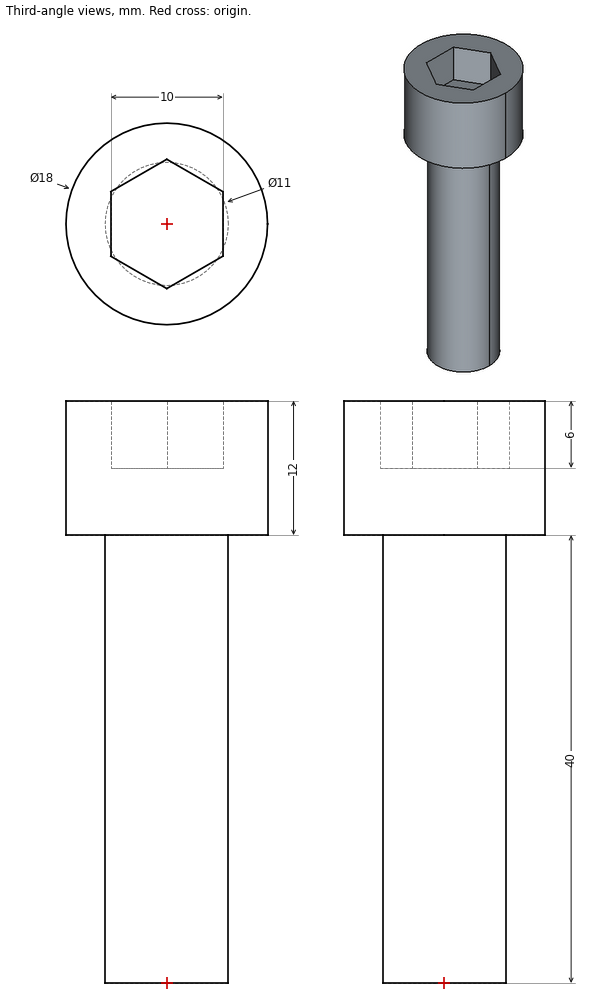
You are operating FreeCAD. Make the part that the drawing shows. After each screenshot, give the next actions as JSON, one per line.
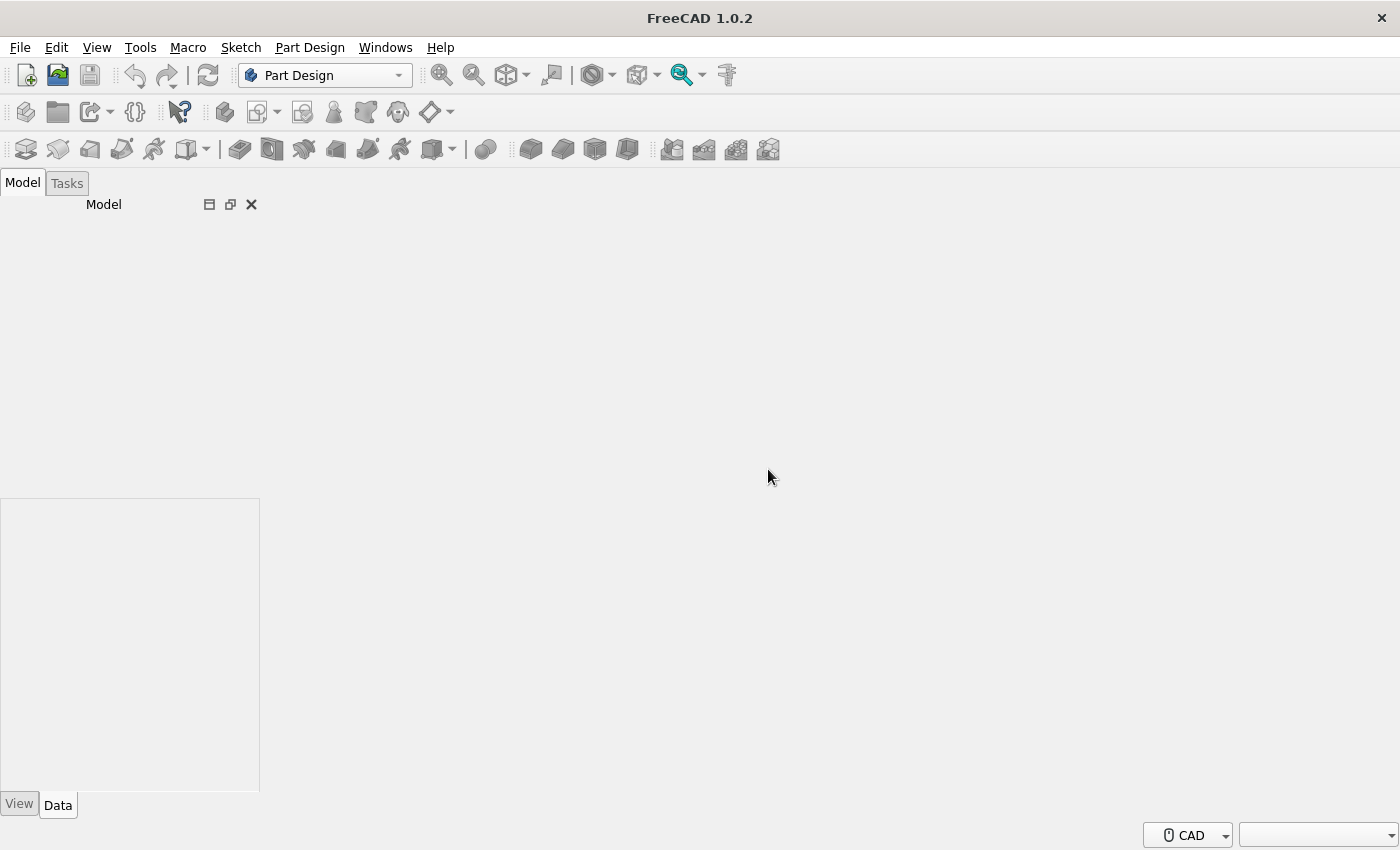
{"action": "left_click", "coordinate": [26, 76]}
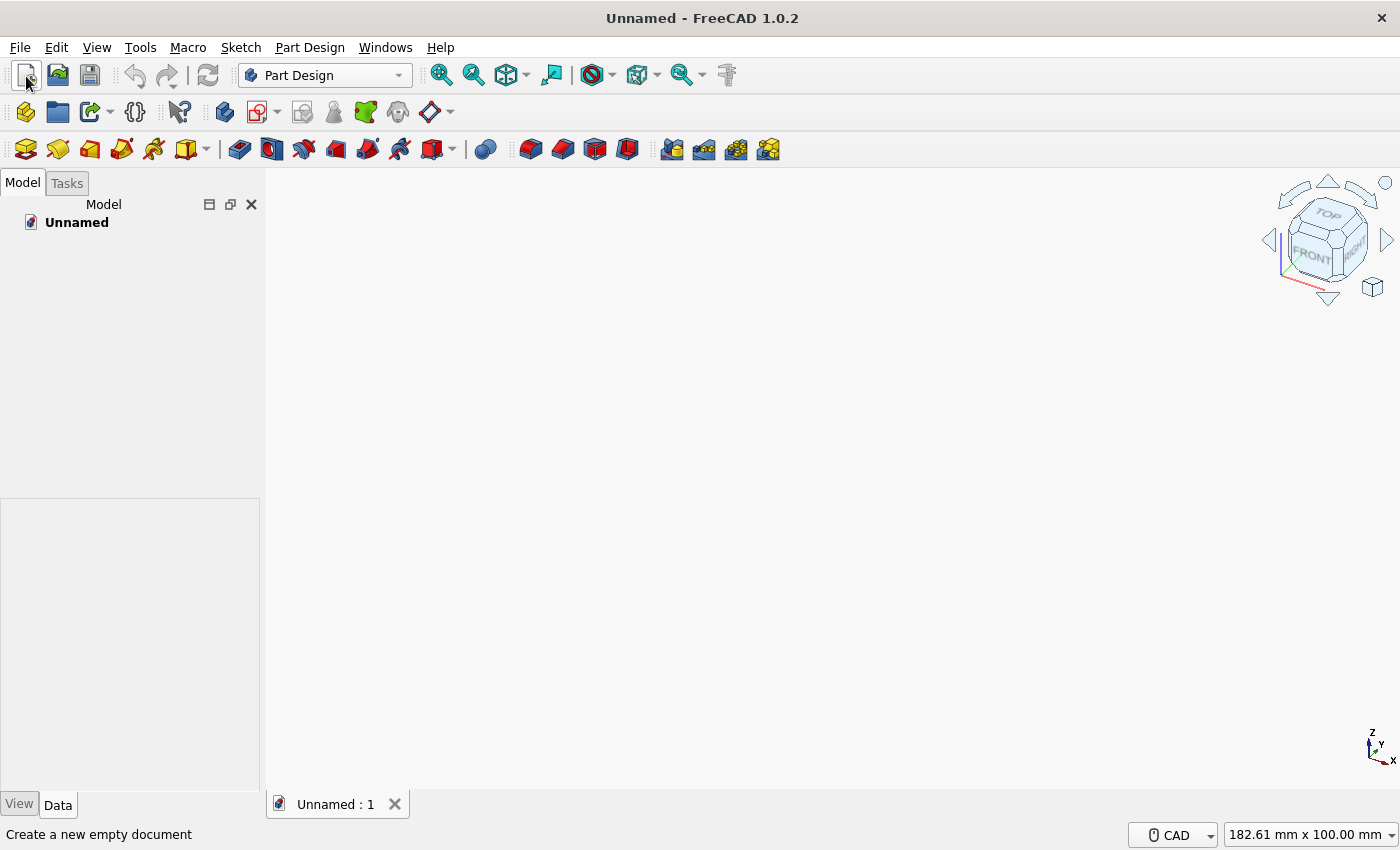
{"action": "left_click", "coordinate": [258, 112]}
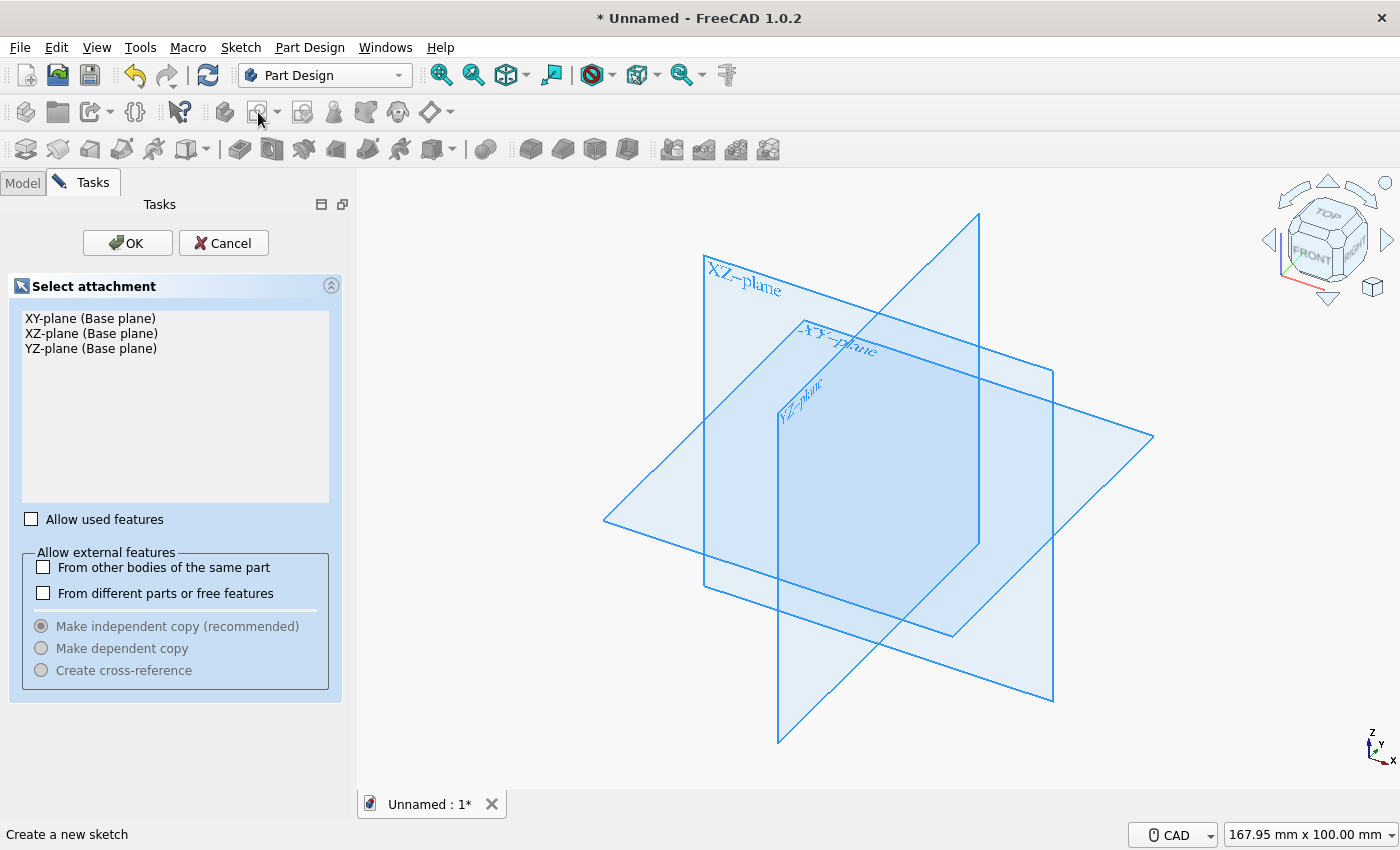
{"action": "left_click", "coordinate": [82, 318]}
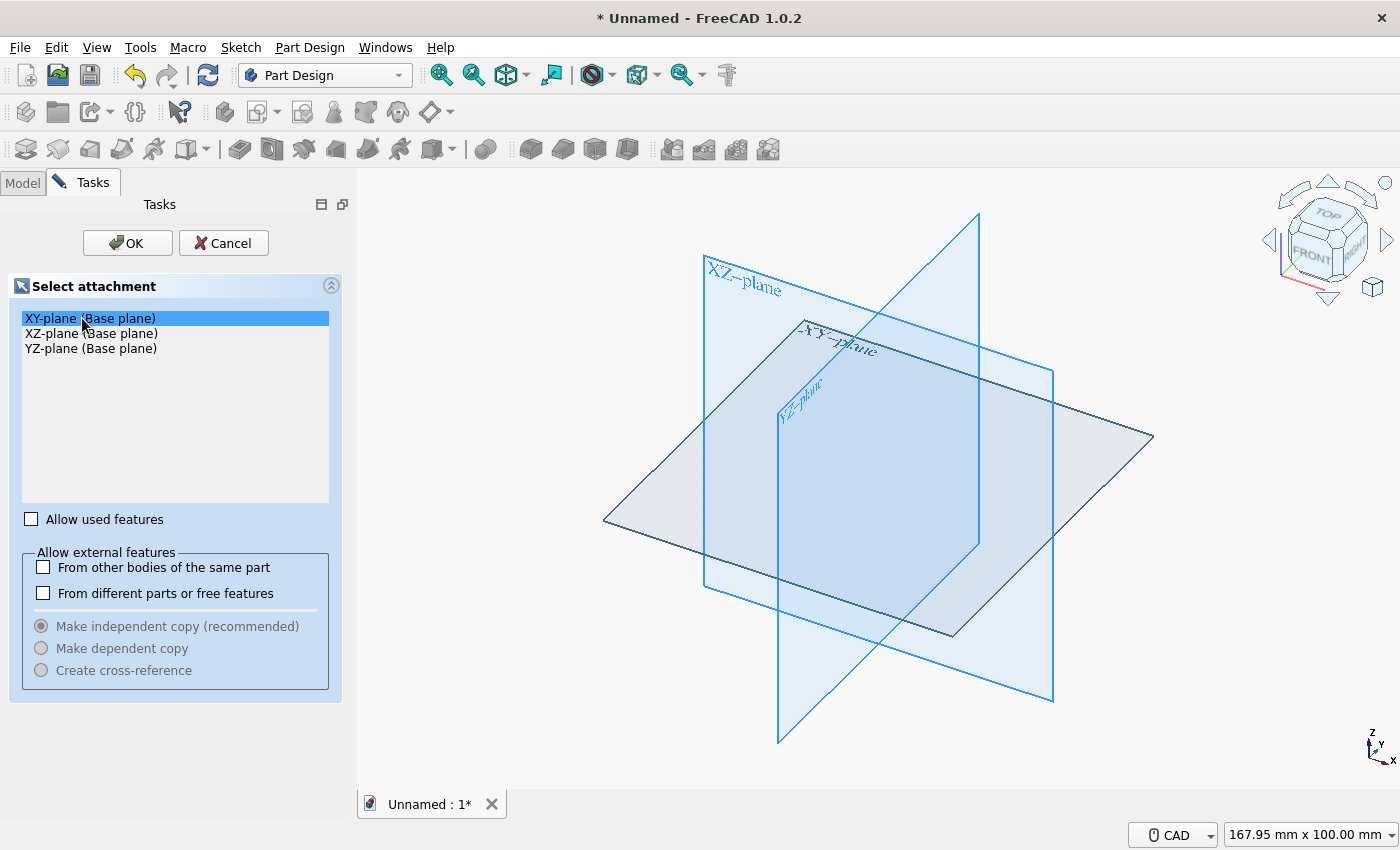
{"action": "left_click", "coordinate": [128, 243]}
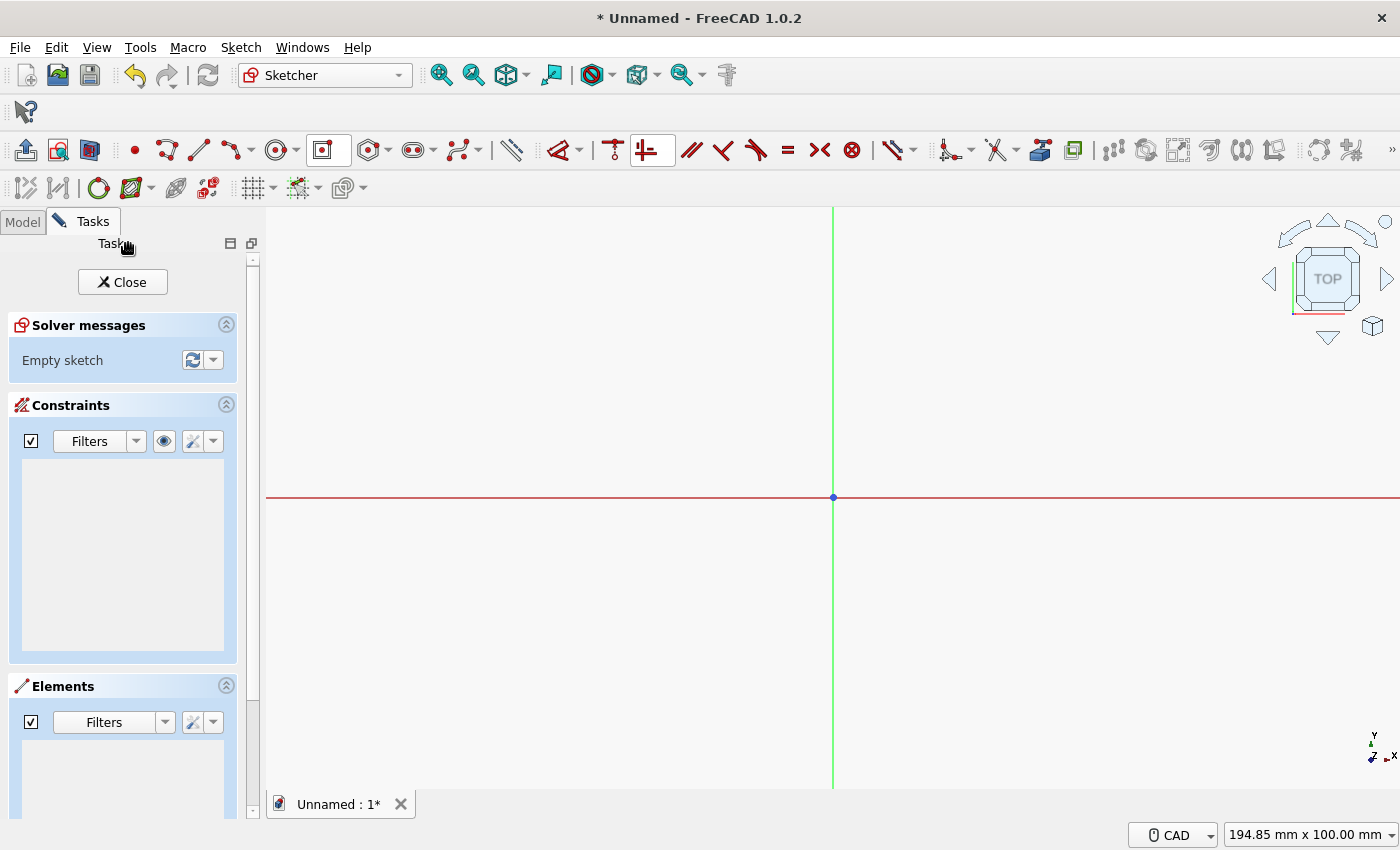
{"action": "scroll", "coordinate": [847, 498], "scroll_direction": "up", "scroll_amount": 9}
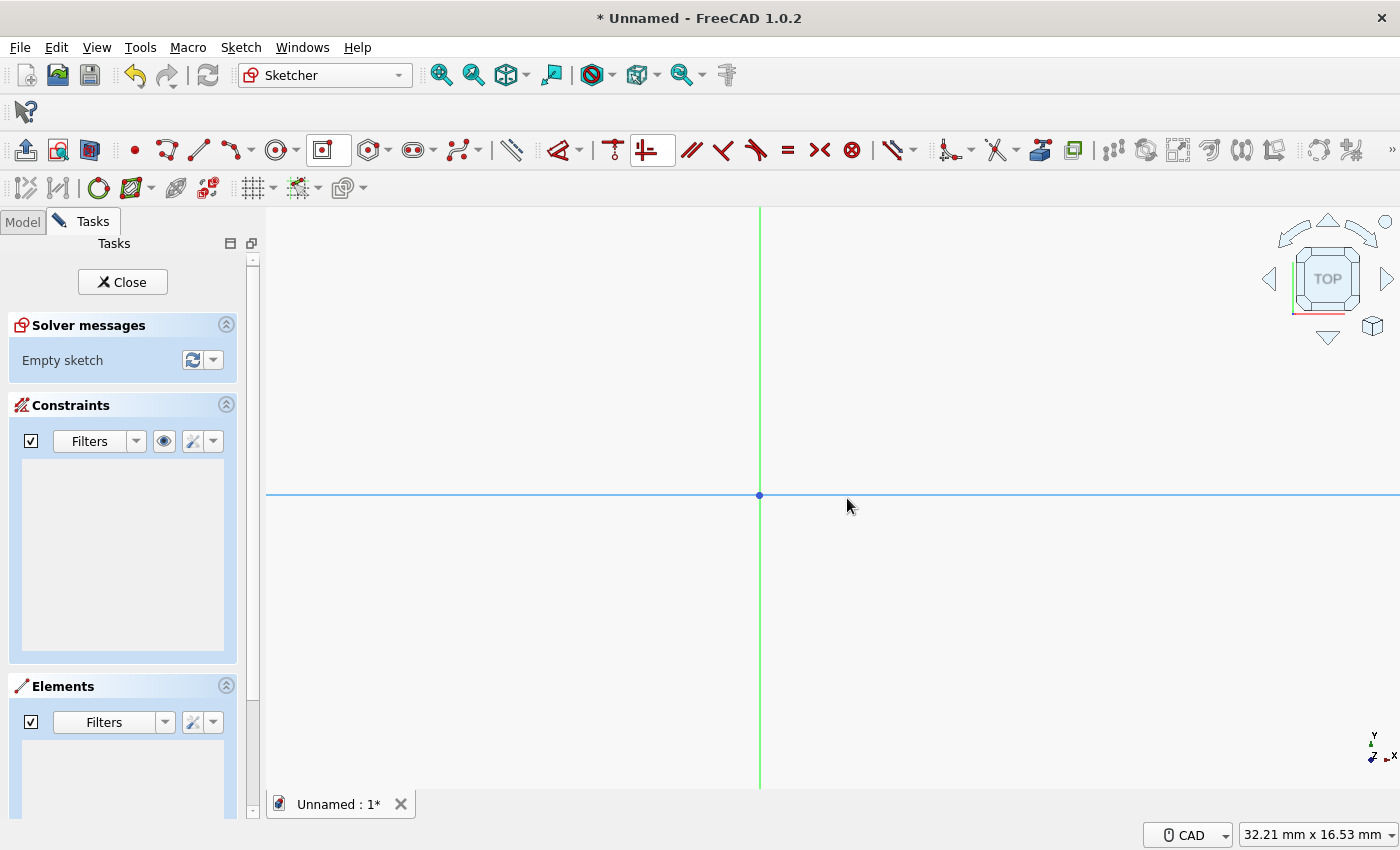
{"action": "left_click", "coordinate": [276, 150]}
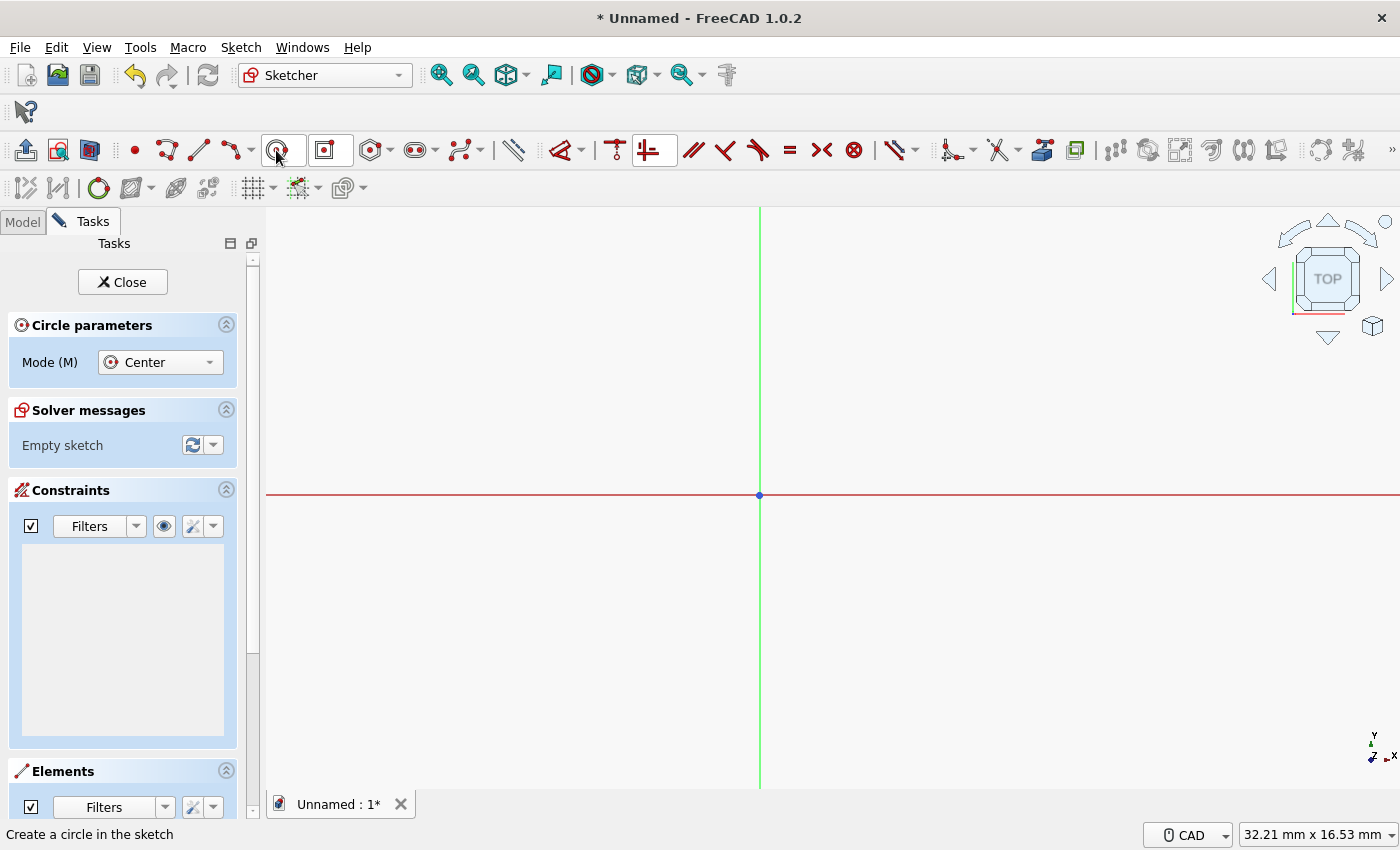
{"action": "left_click", "coordinate": [760, 495]}
{"action": "mouse_move", "coordinate": [897, 359]}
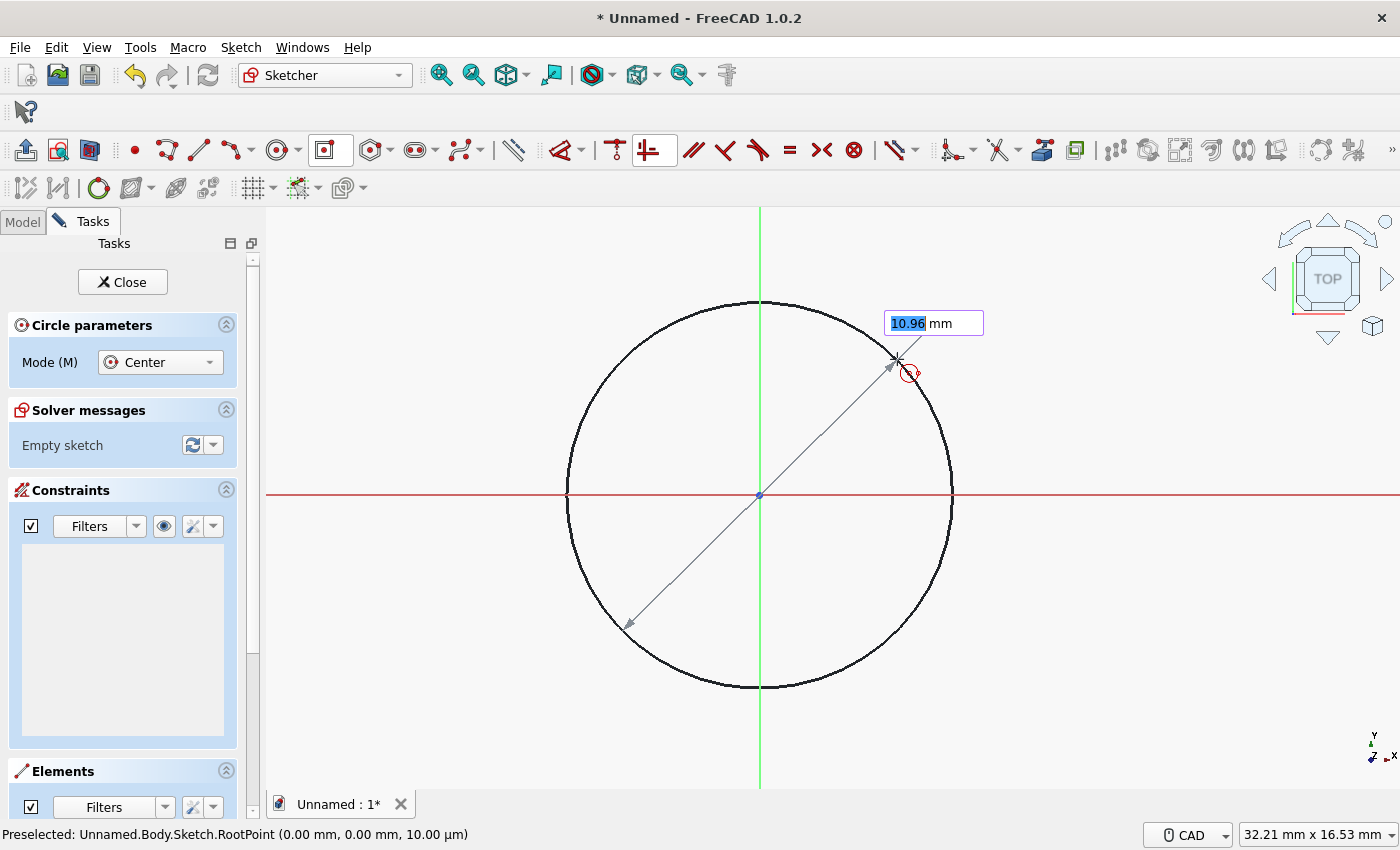
{"action": "type", "text": "11"}
{"action": "key", "text": "Return"}
{"action": "key", "text": "Escape"}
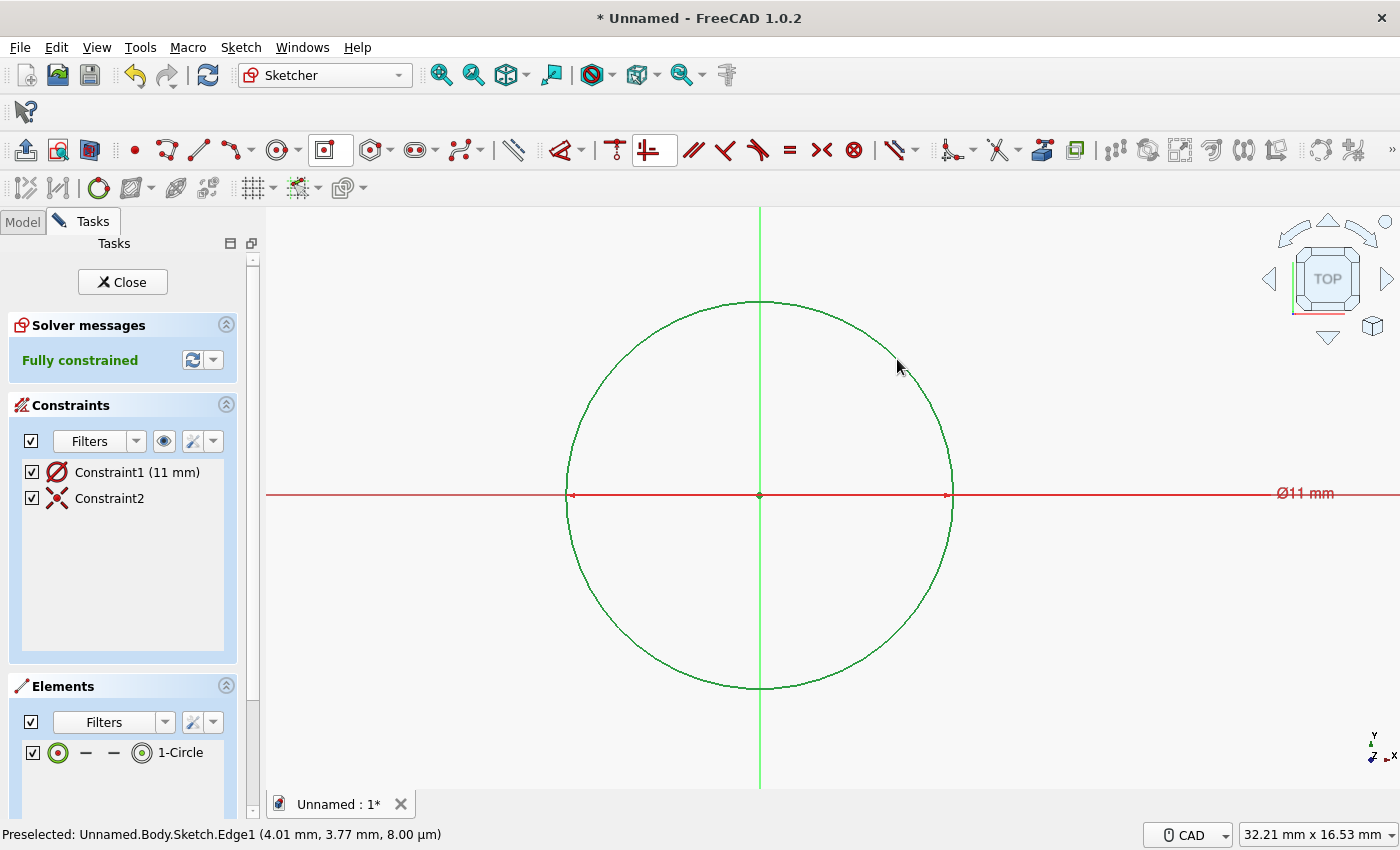
{"action": "left_click", "coordinate": [123, 282]}